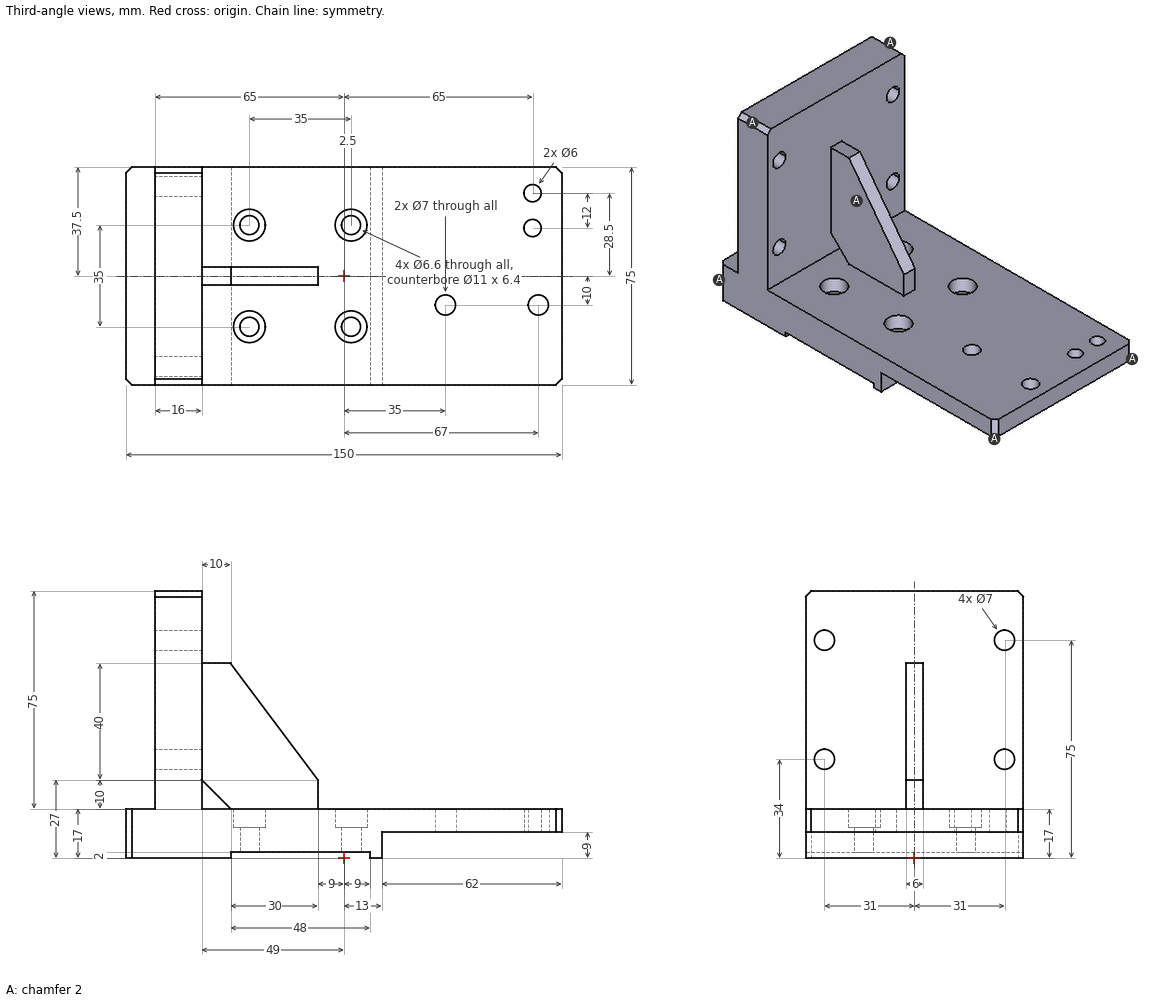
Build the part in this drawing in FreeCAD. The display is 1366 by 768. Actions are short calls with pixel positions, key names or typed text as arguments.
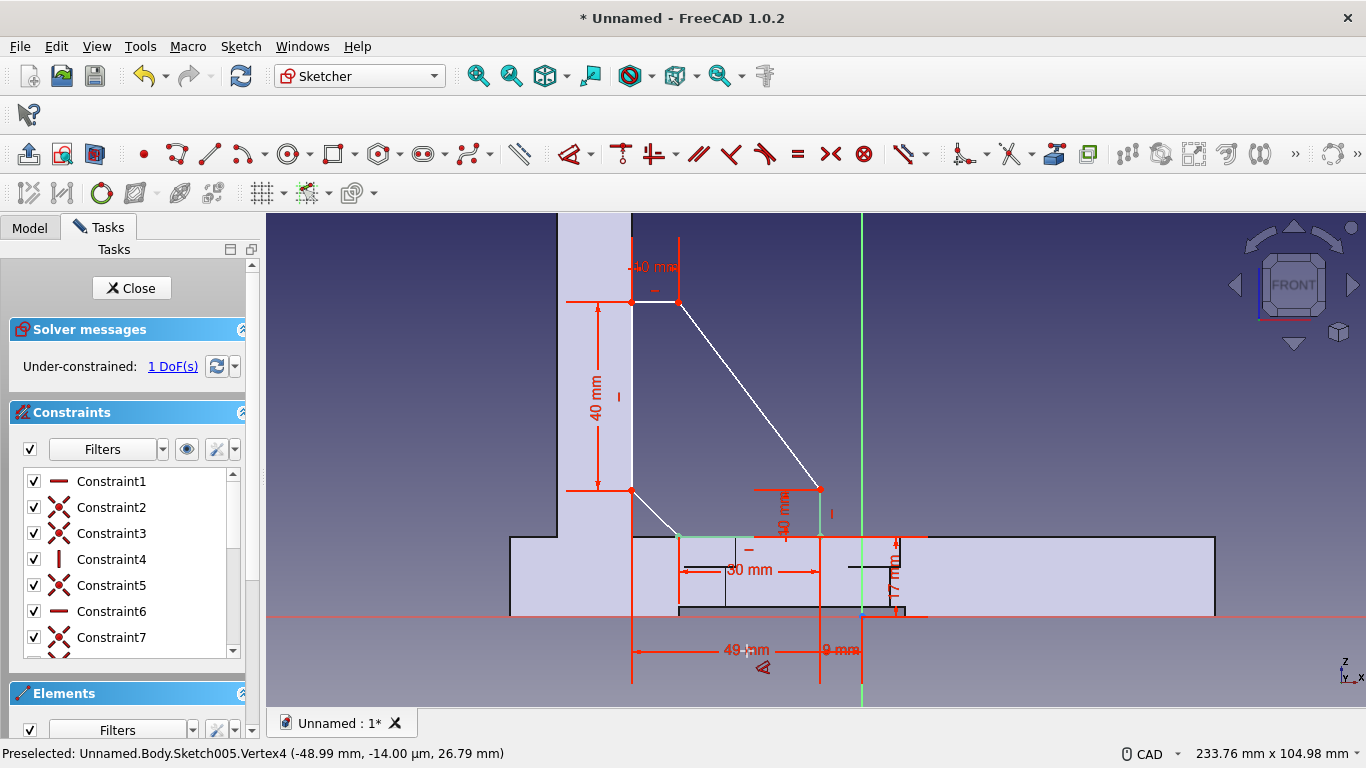
click(632, 491)
click(896, 554)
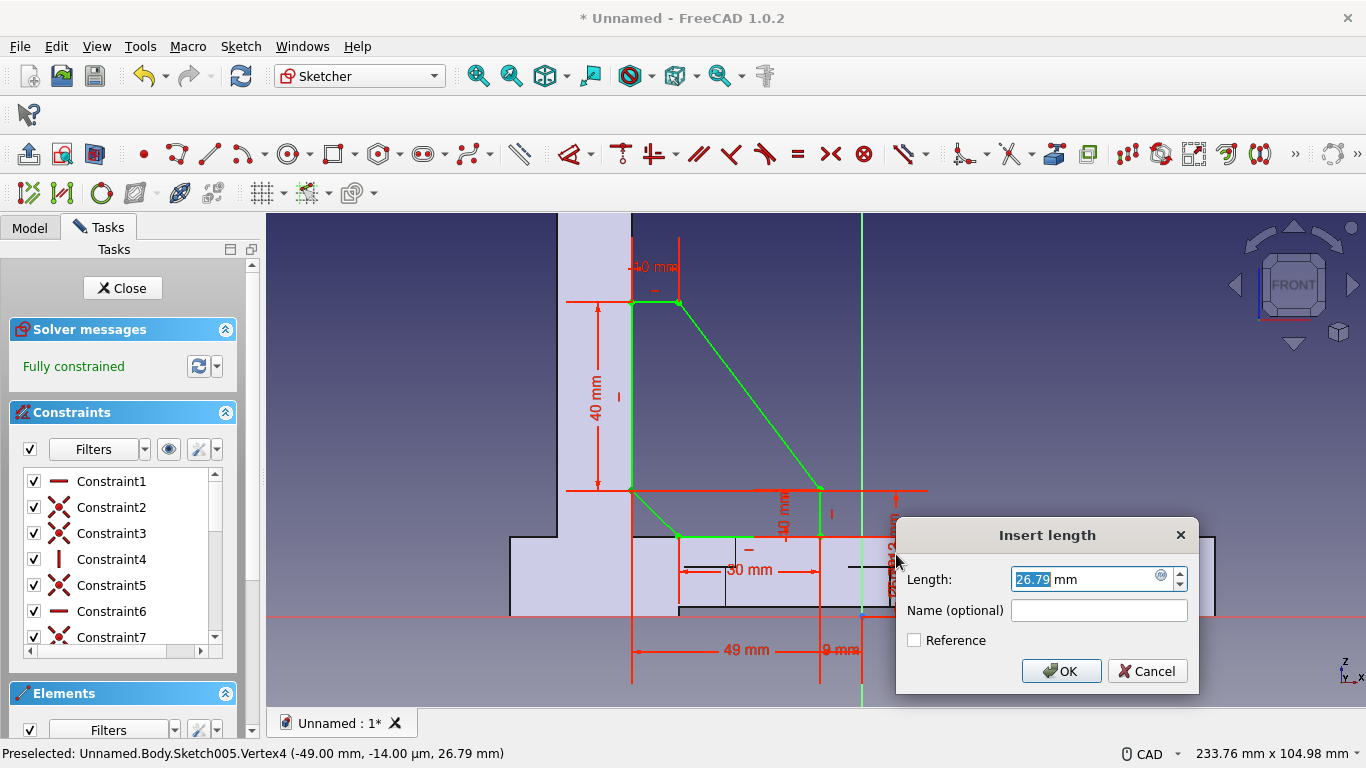
text(27)
key(Return)
key(Escape)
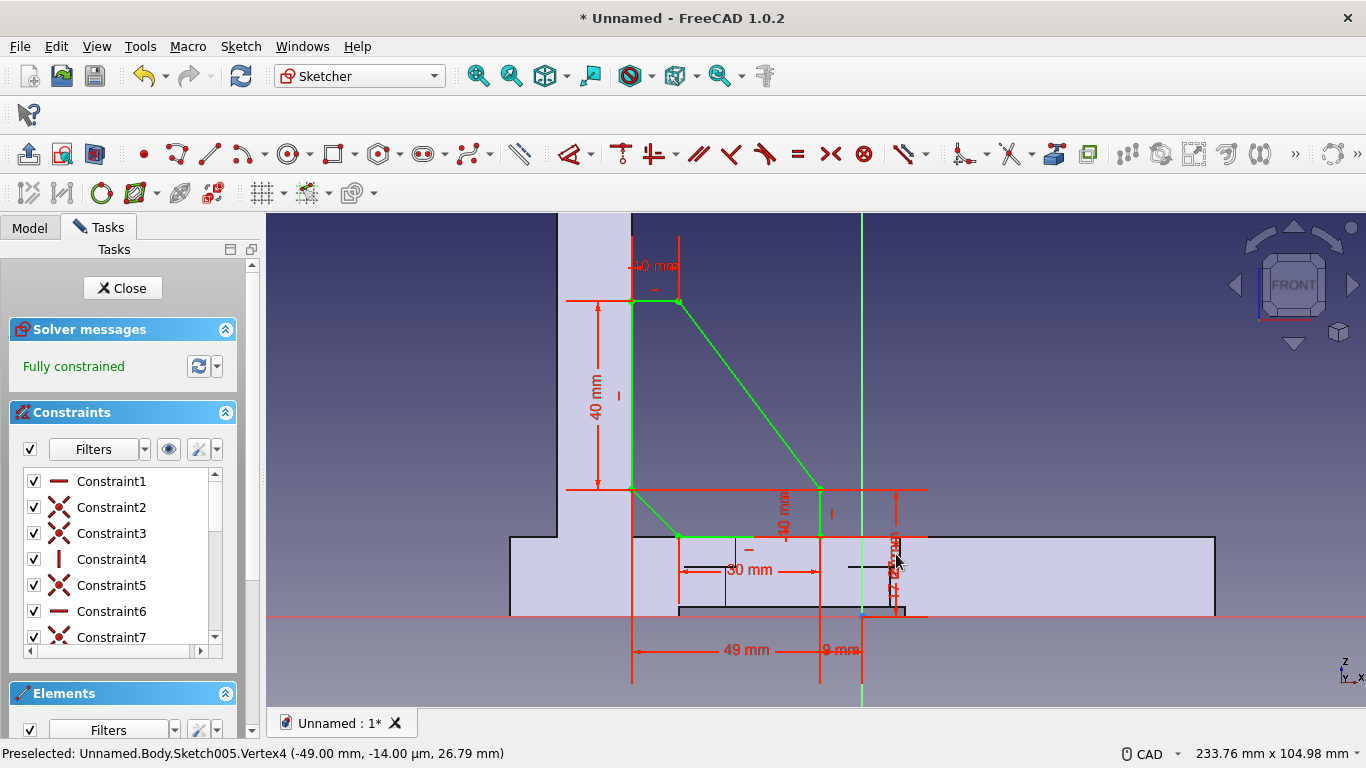
click(123, 288)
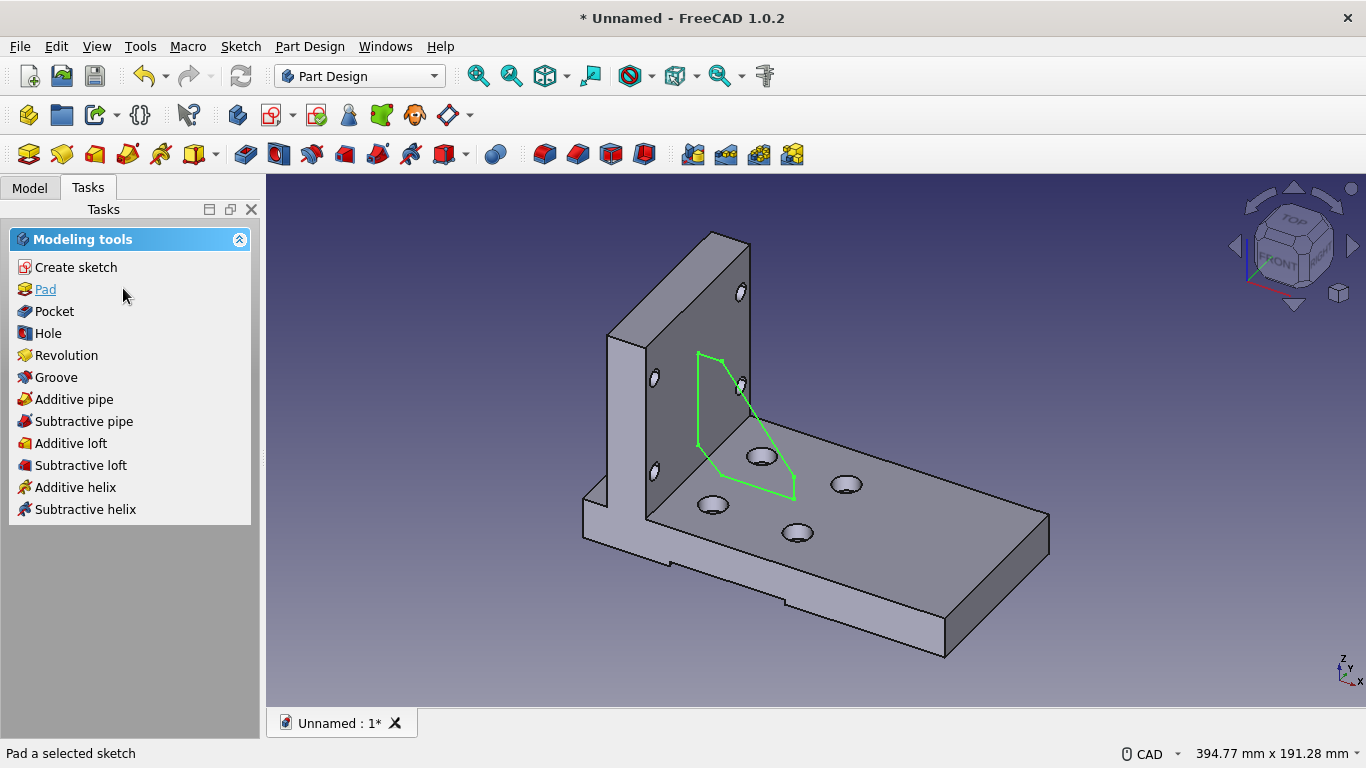
click(29, 154)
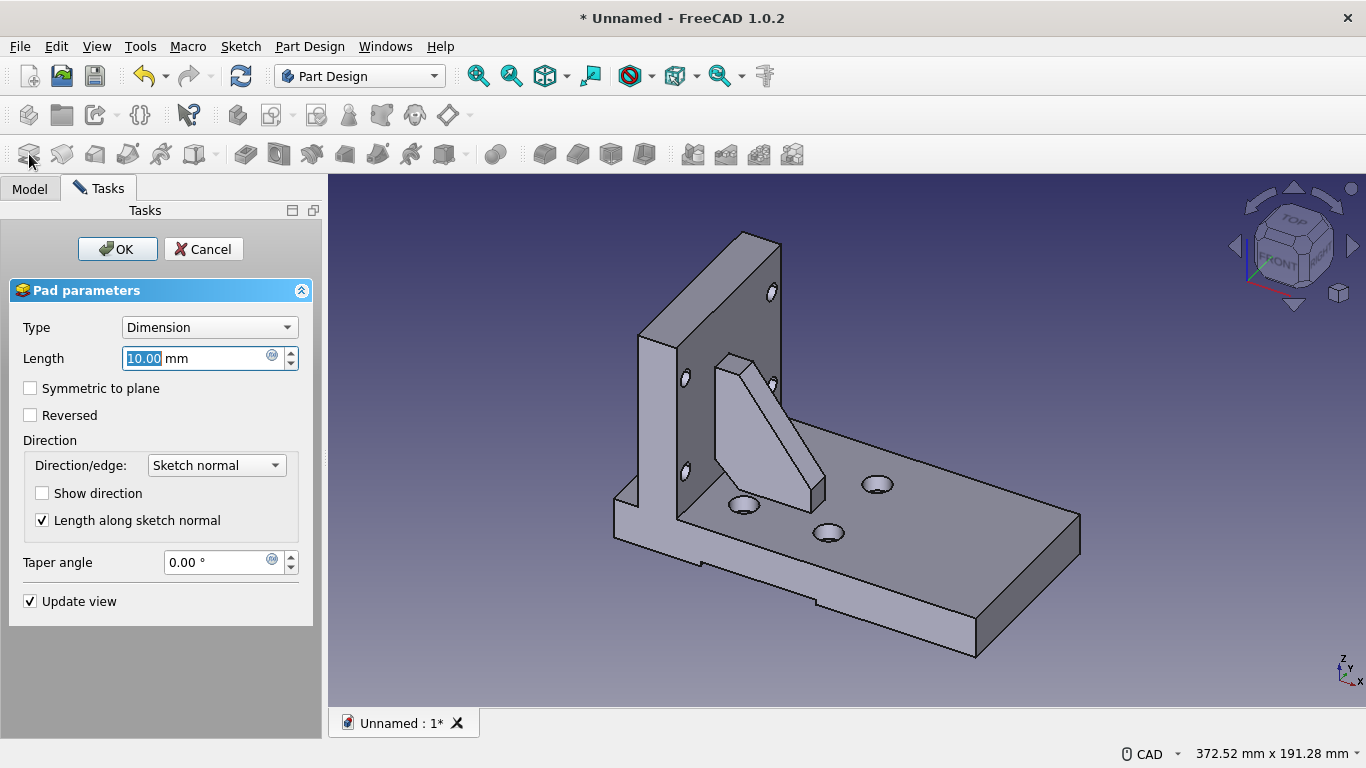
text(6)
key(Tab)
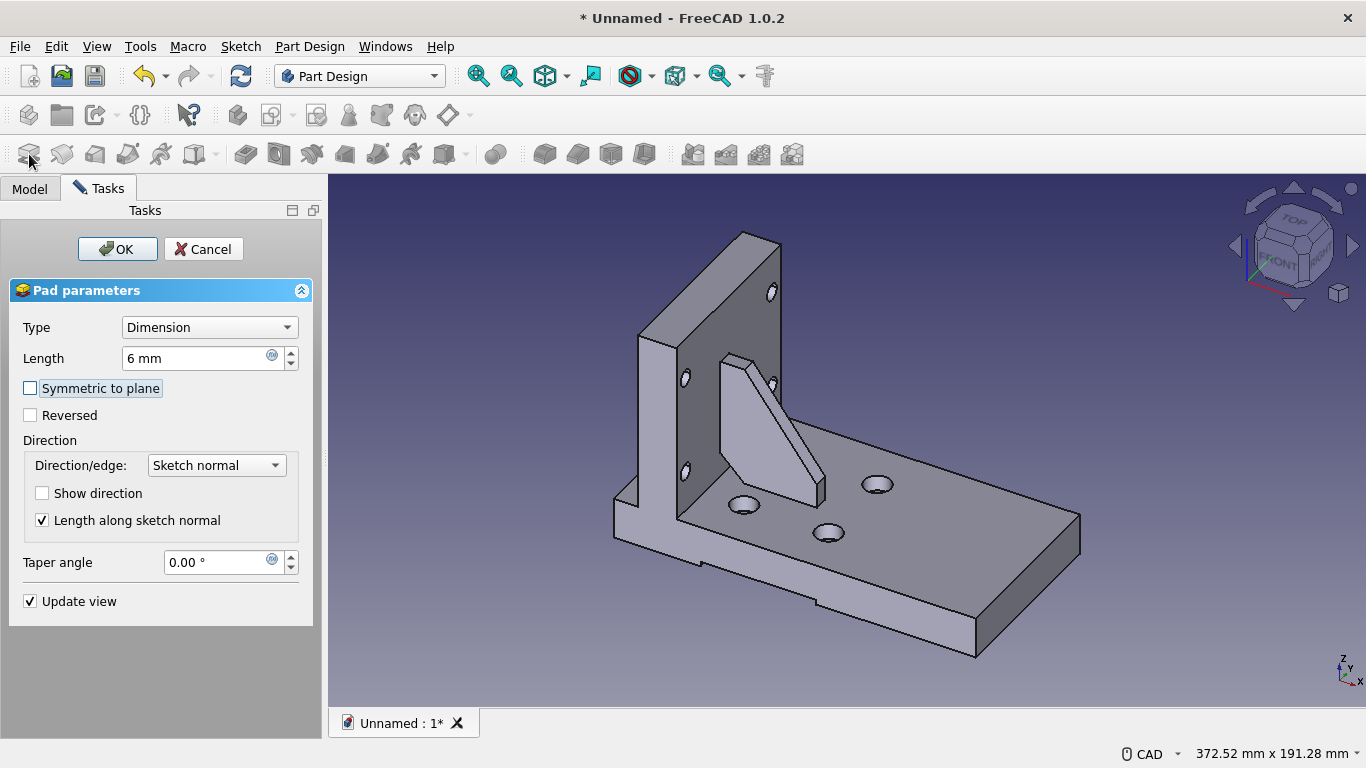
click(31, 388)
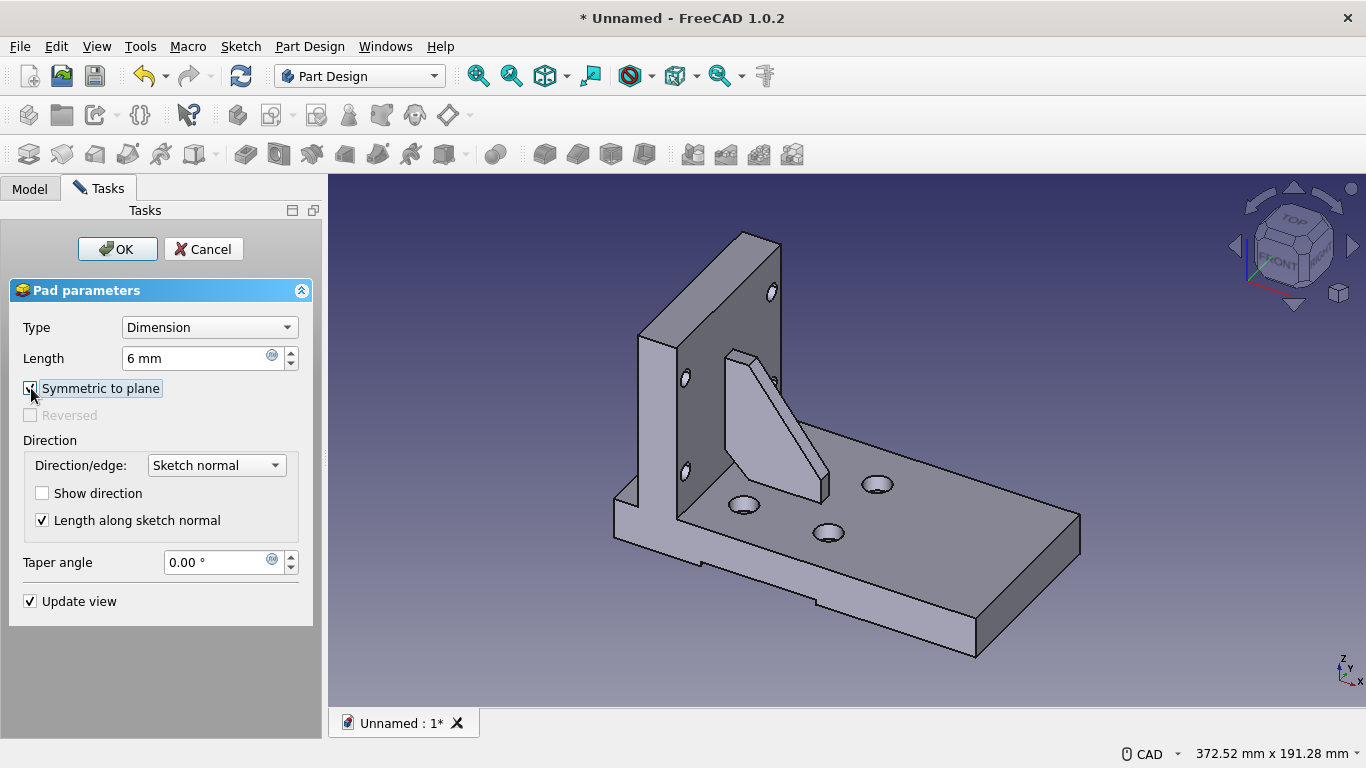
click(118, 249)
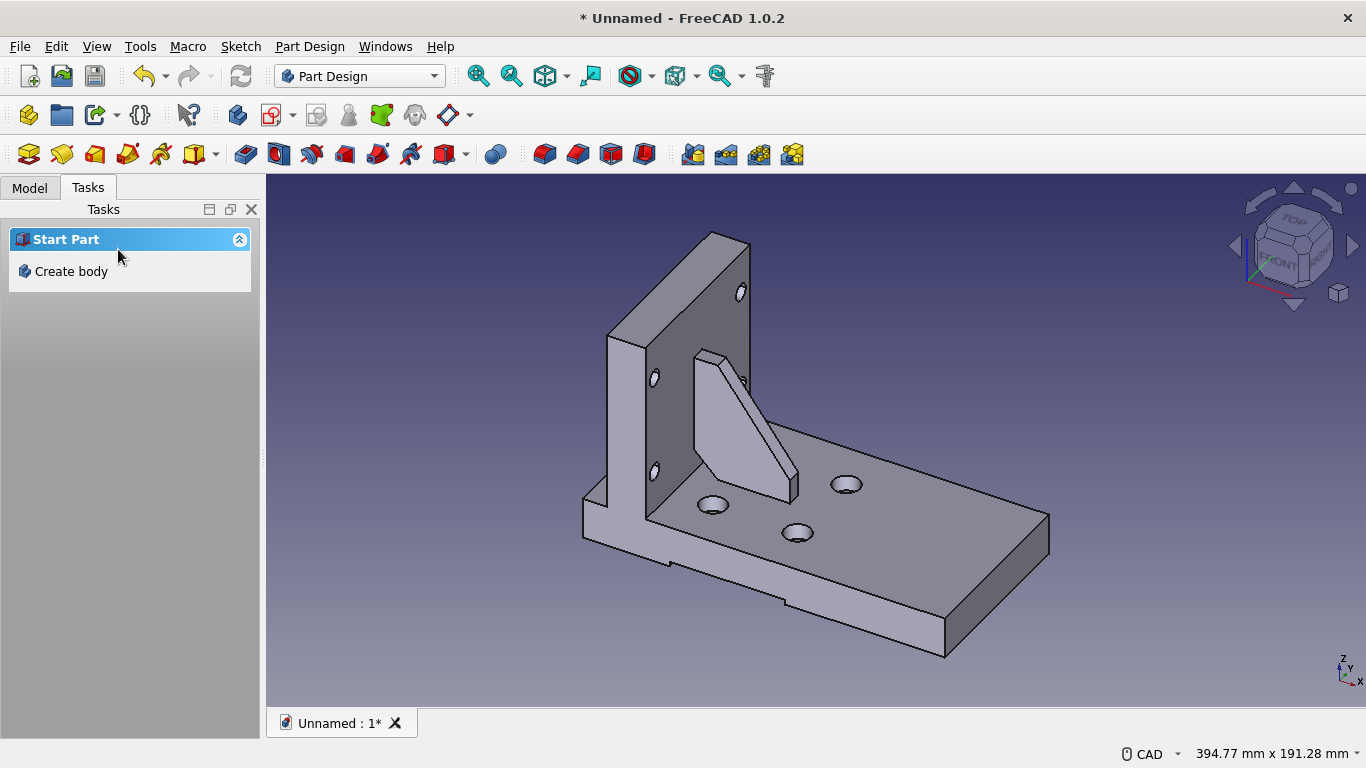
click(945, 637)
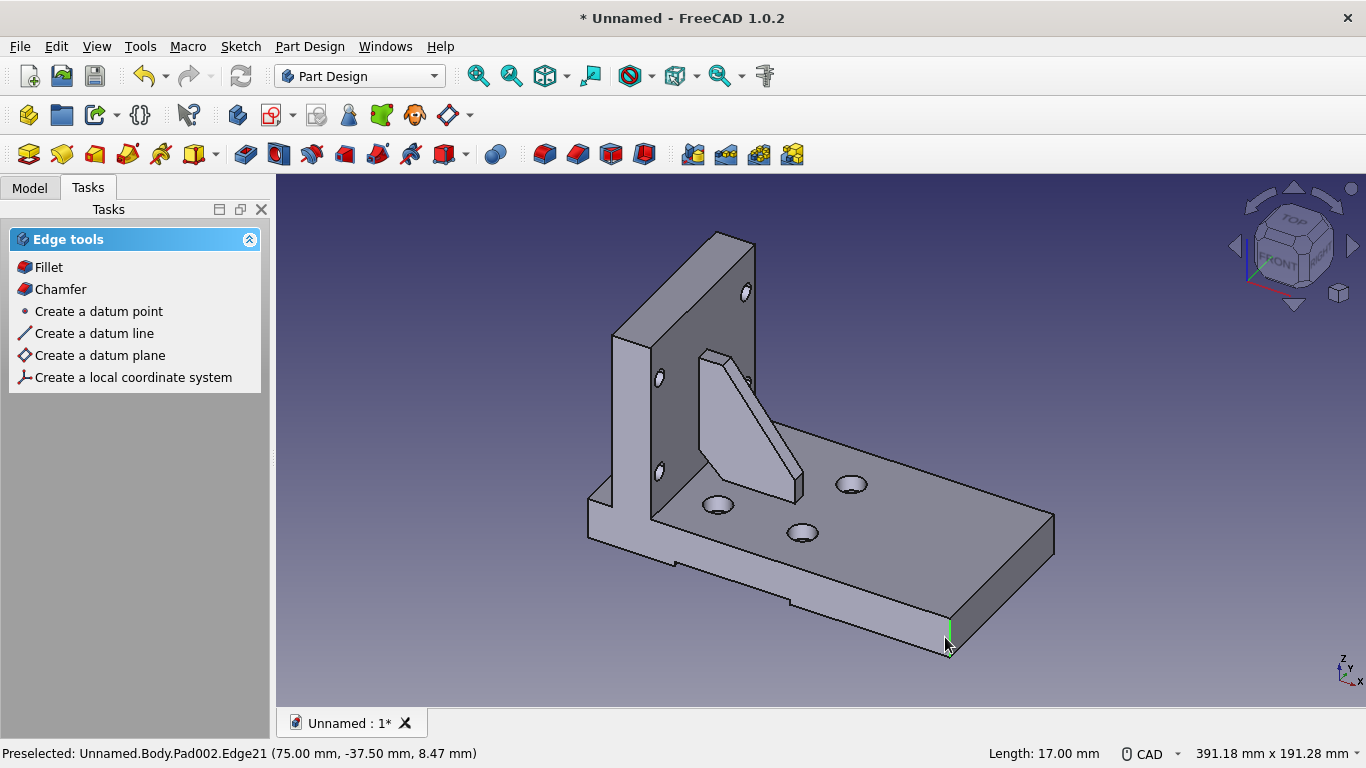
click(631, 341, ctrl)